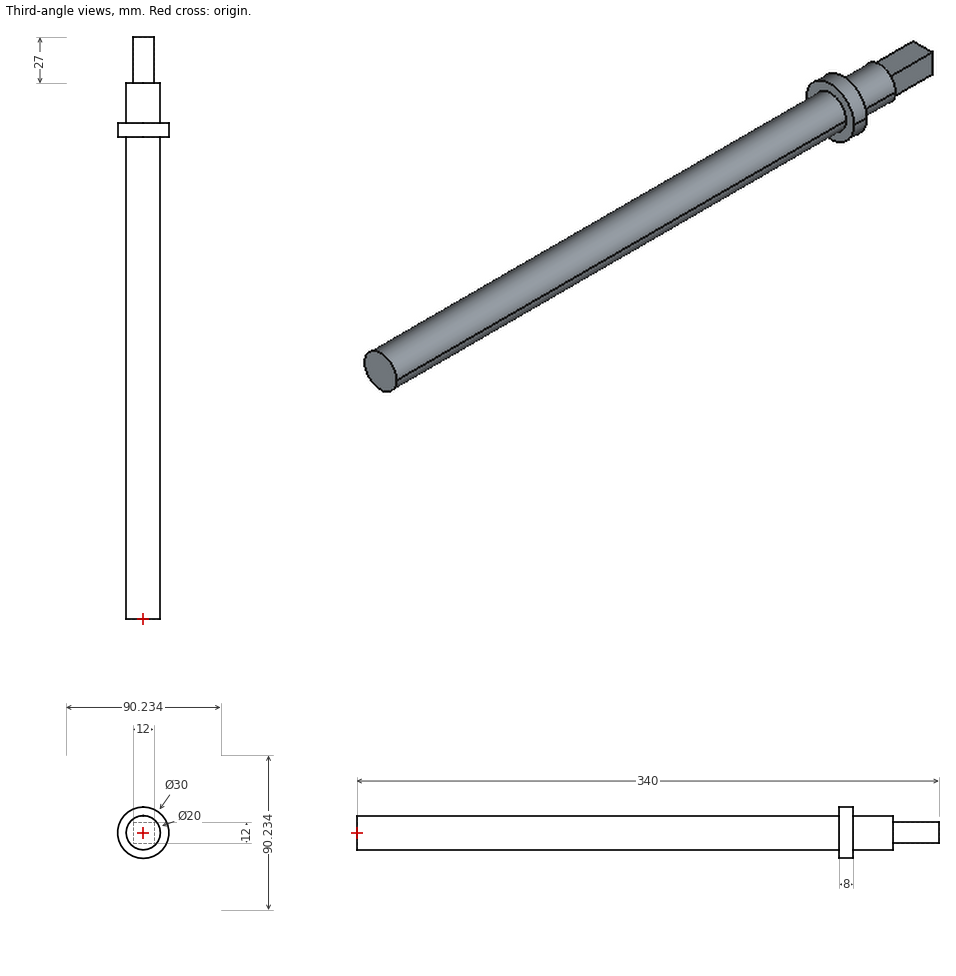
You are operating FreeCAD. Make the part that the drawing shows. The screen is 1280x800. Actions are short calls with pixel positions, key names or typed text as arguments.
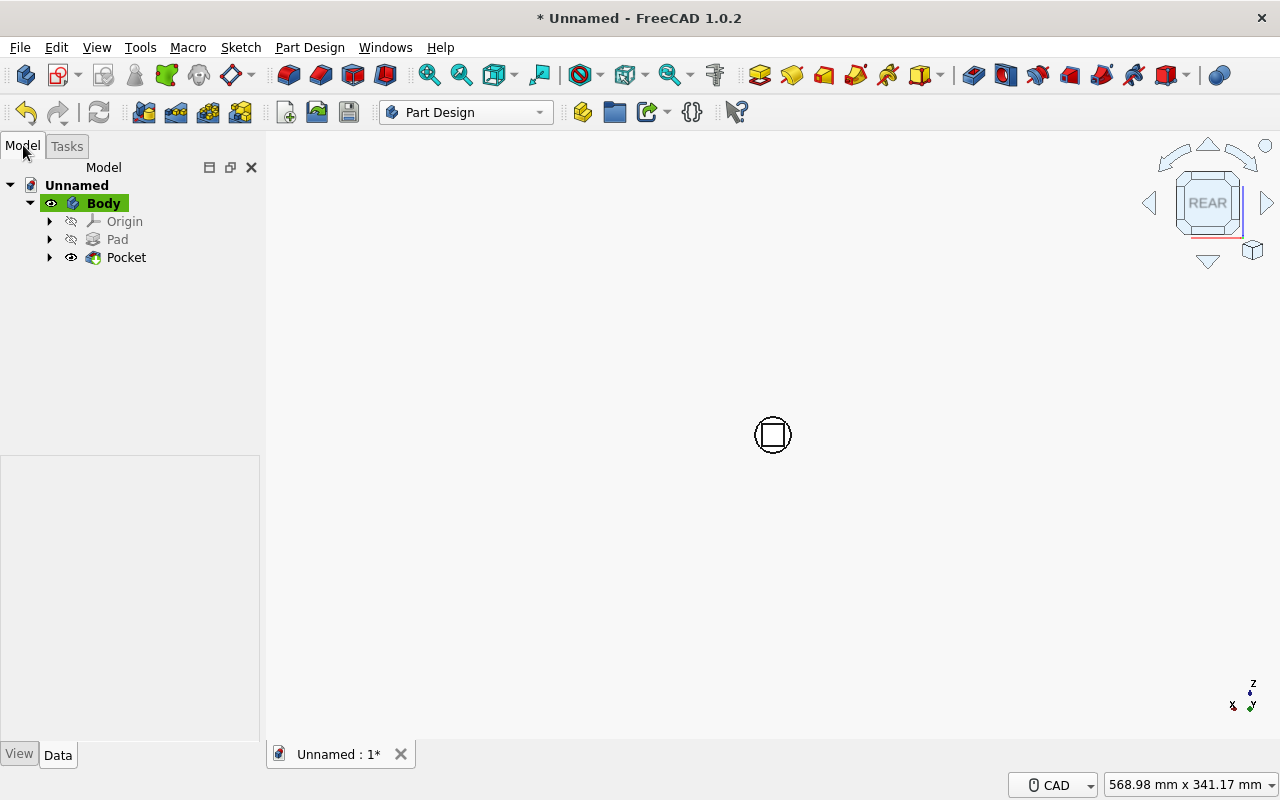
click(50, 221)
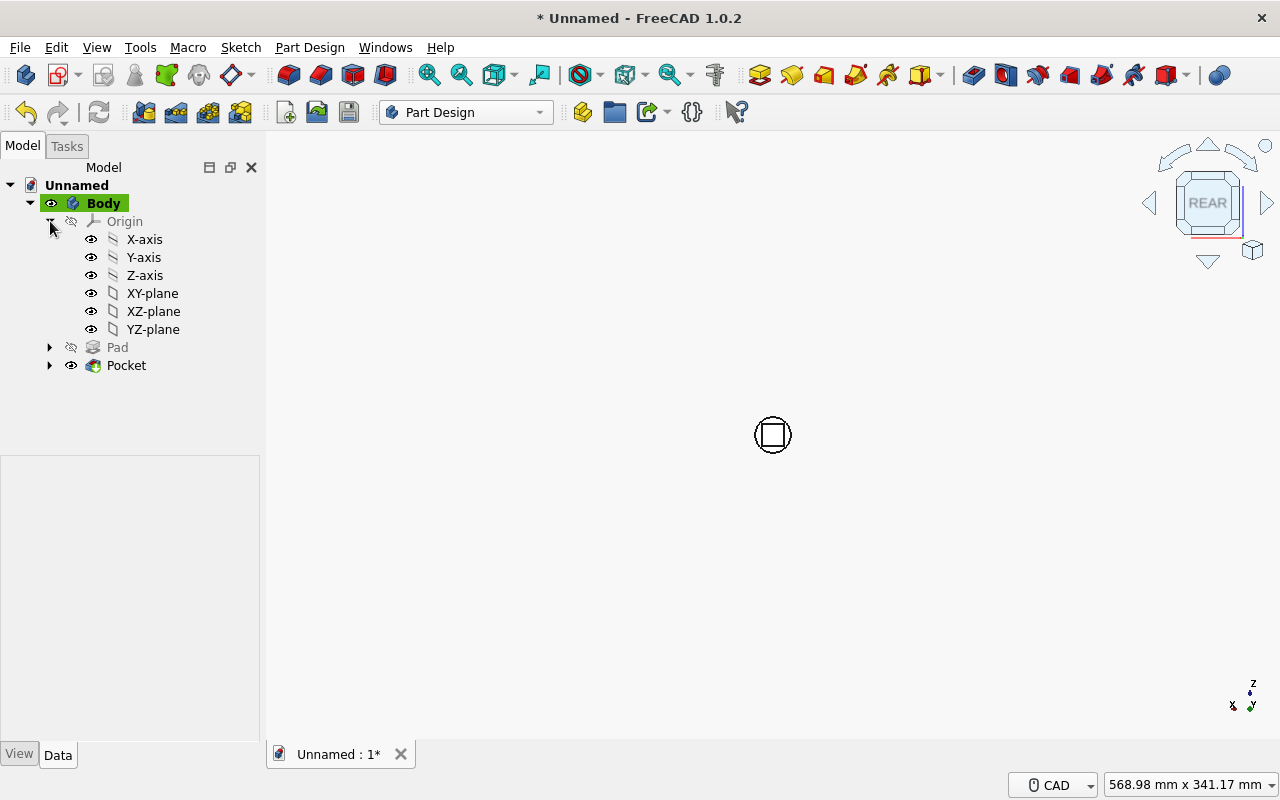
click(136, 311)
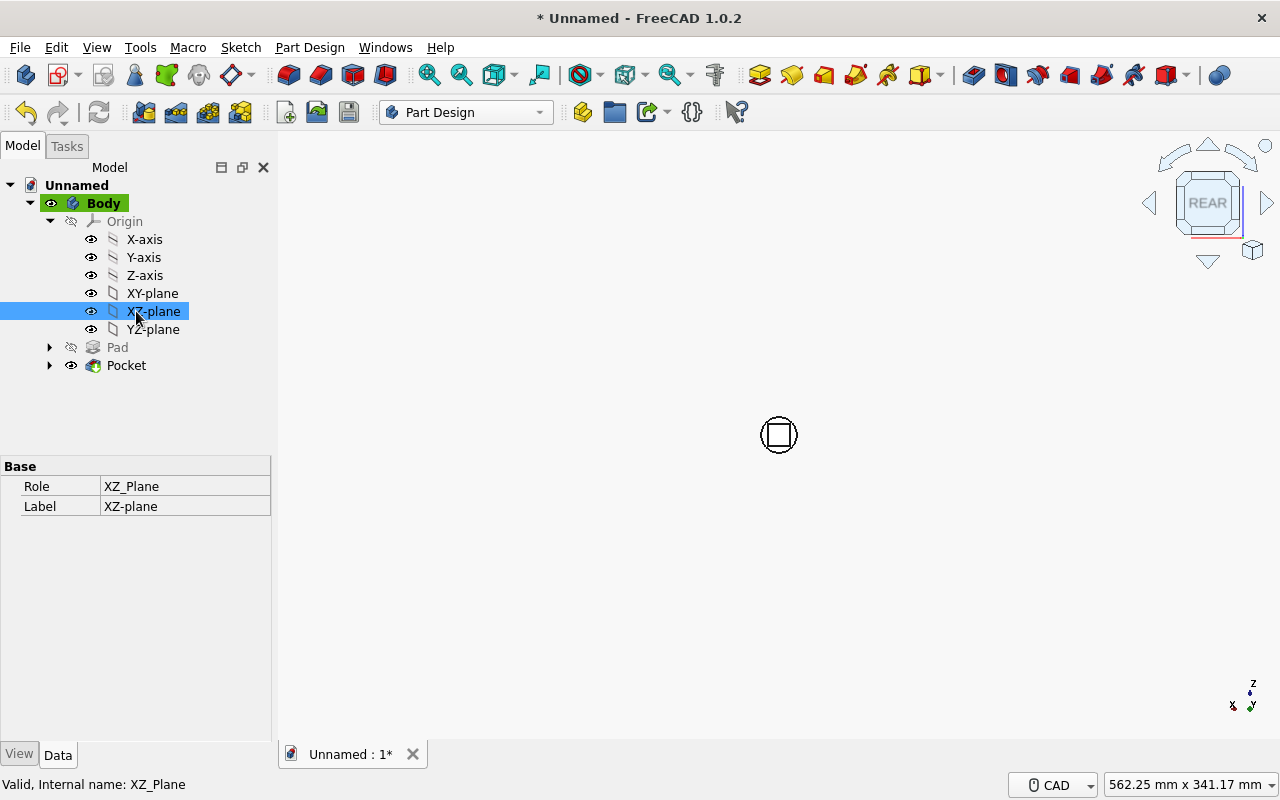
click(232, 76)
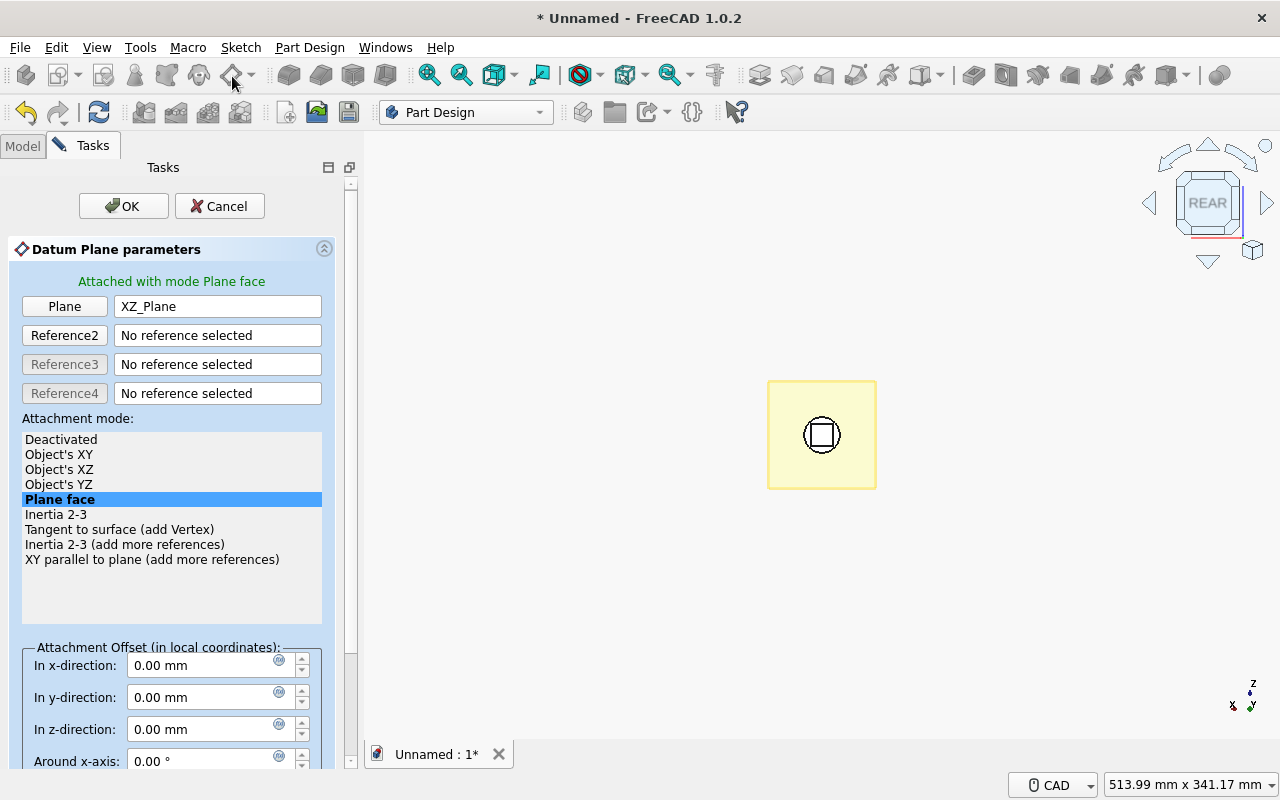
triple_click(210, 729)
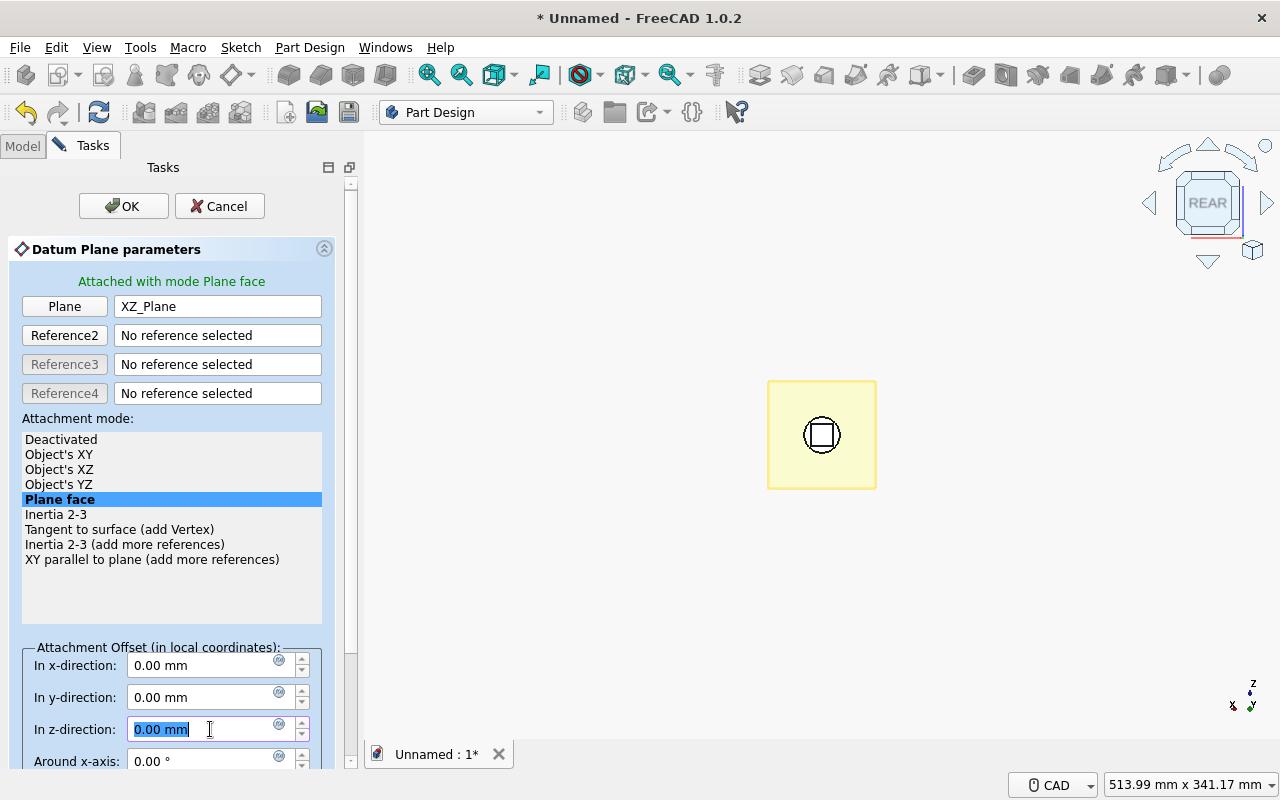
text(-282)
key(Tab)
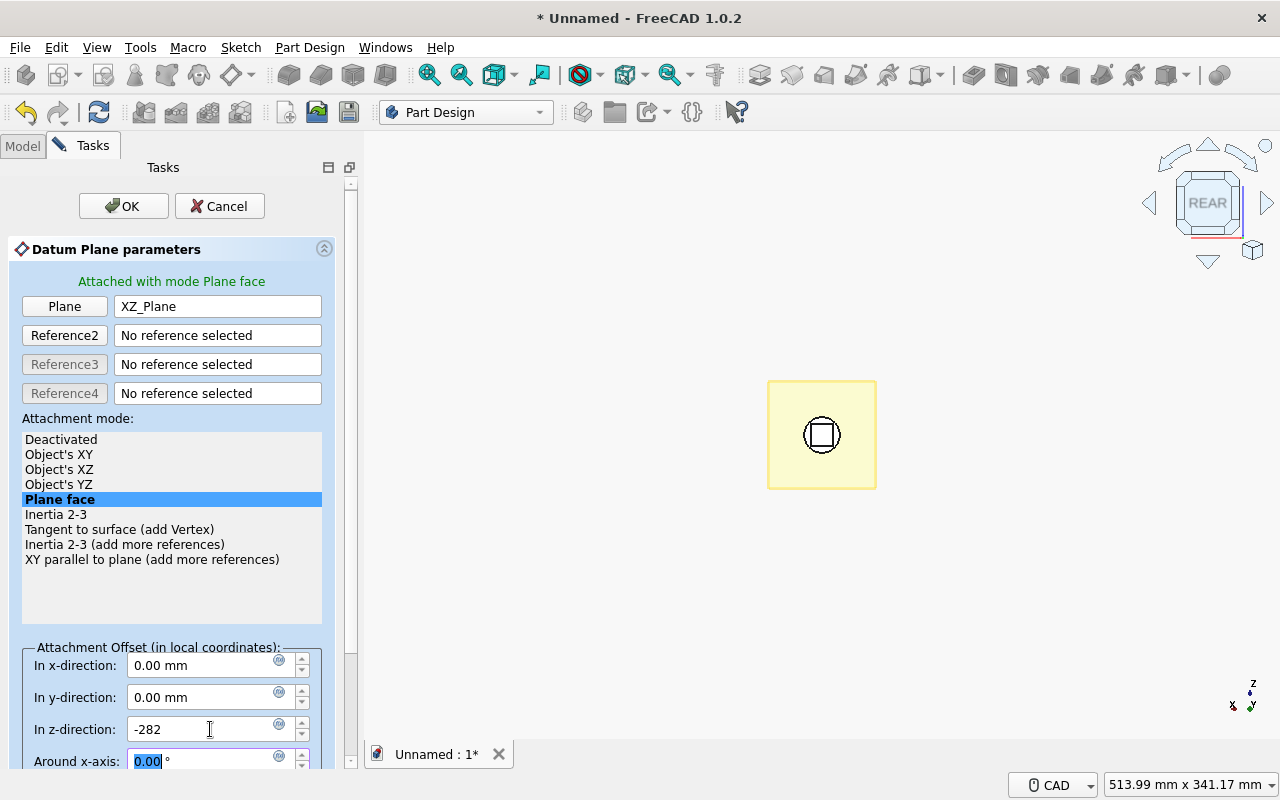
click(124, 206)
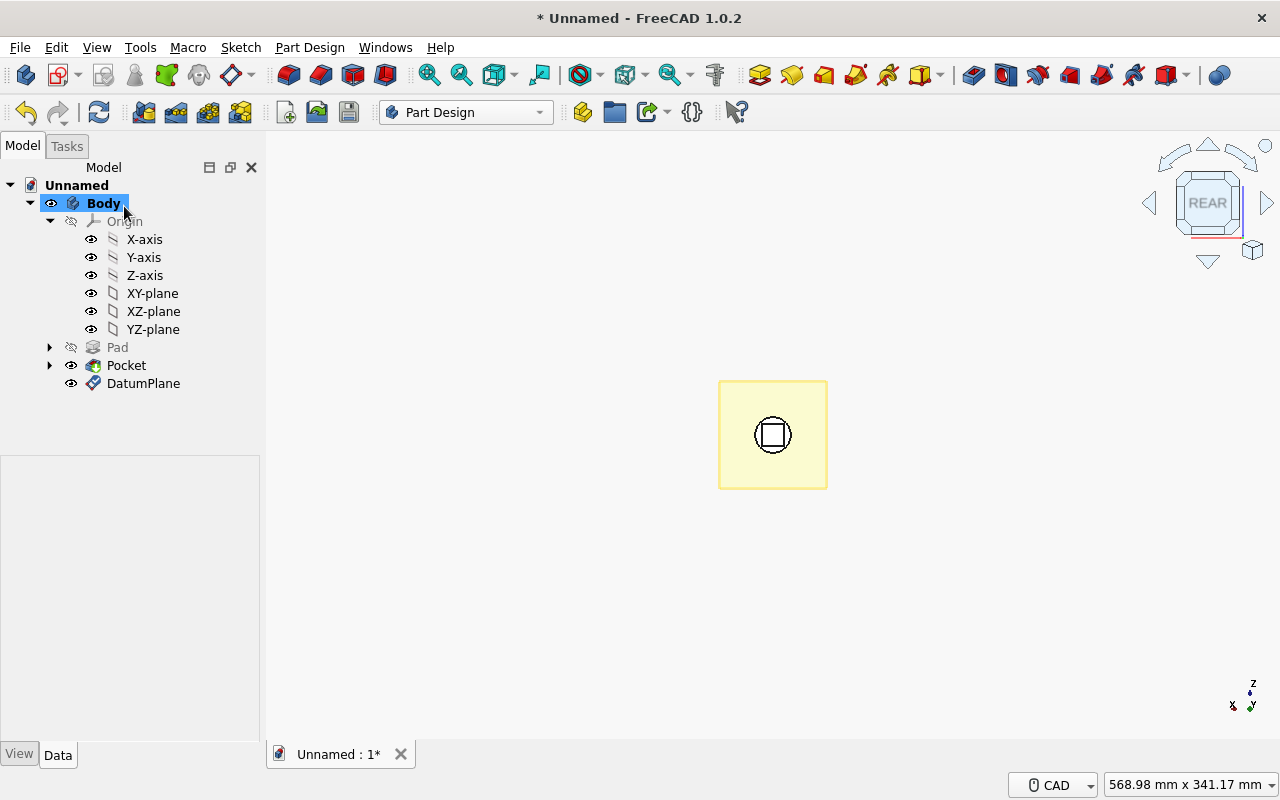
click(116, 383)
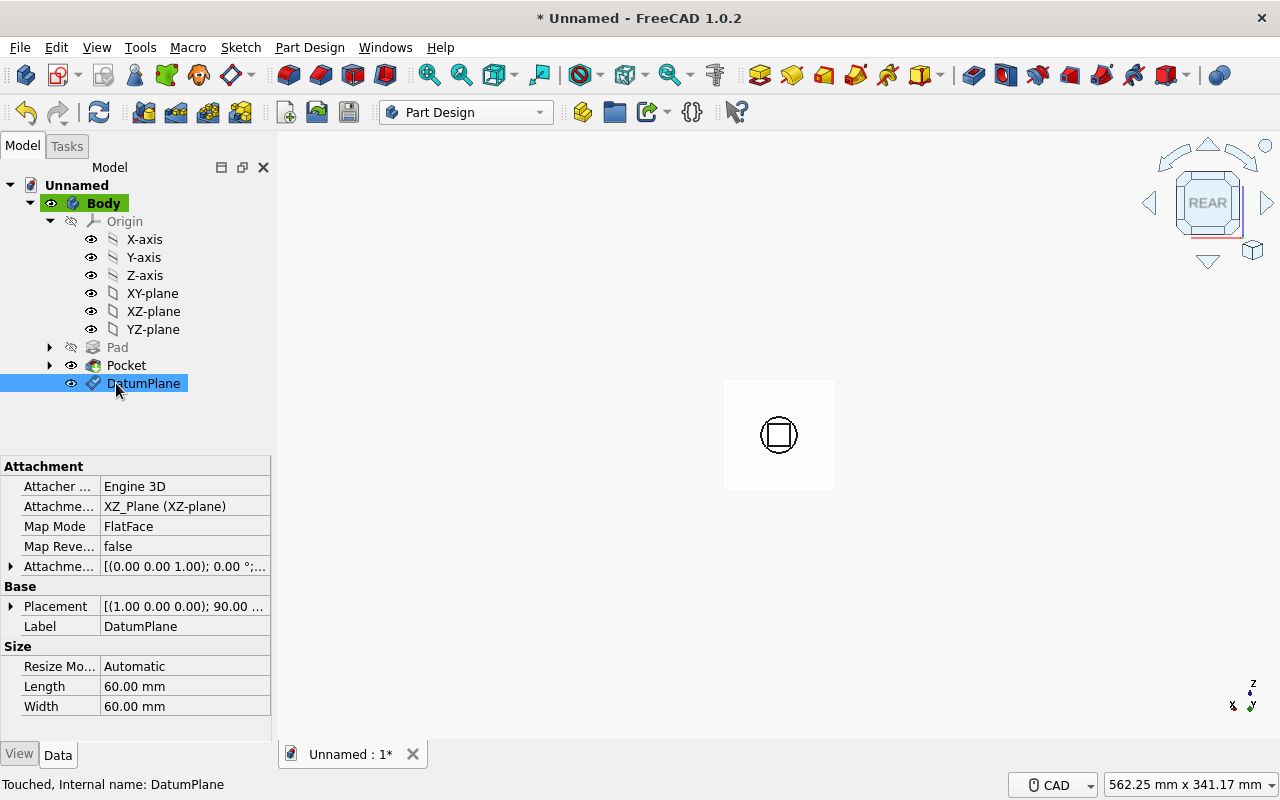
click(58, 76)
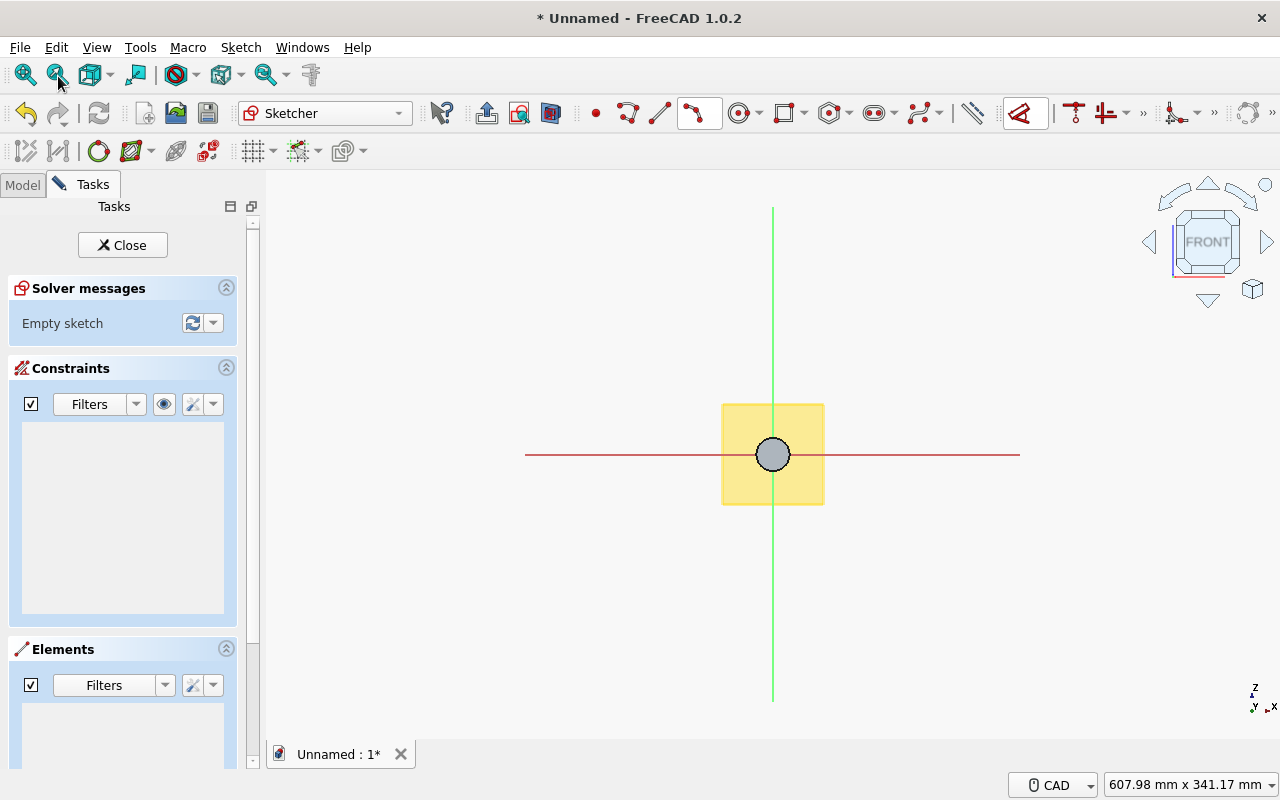
click(552, 114)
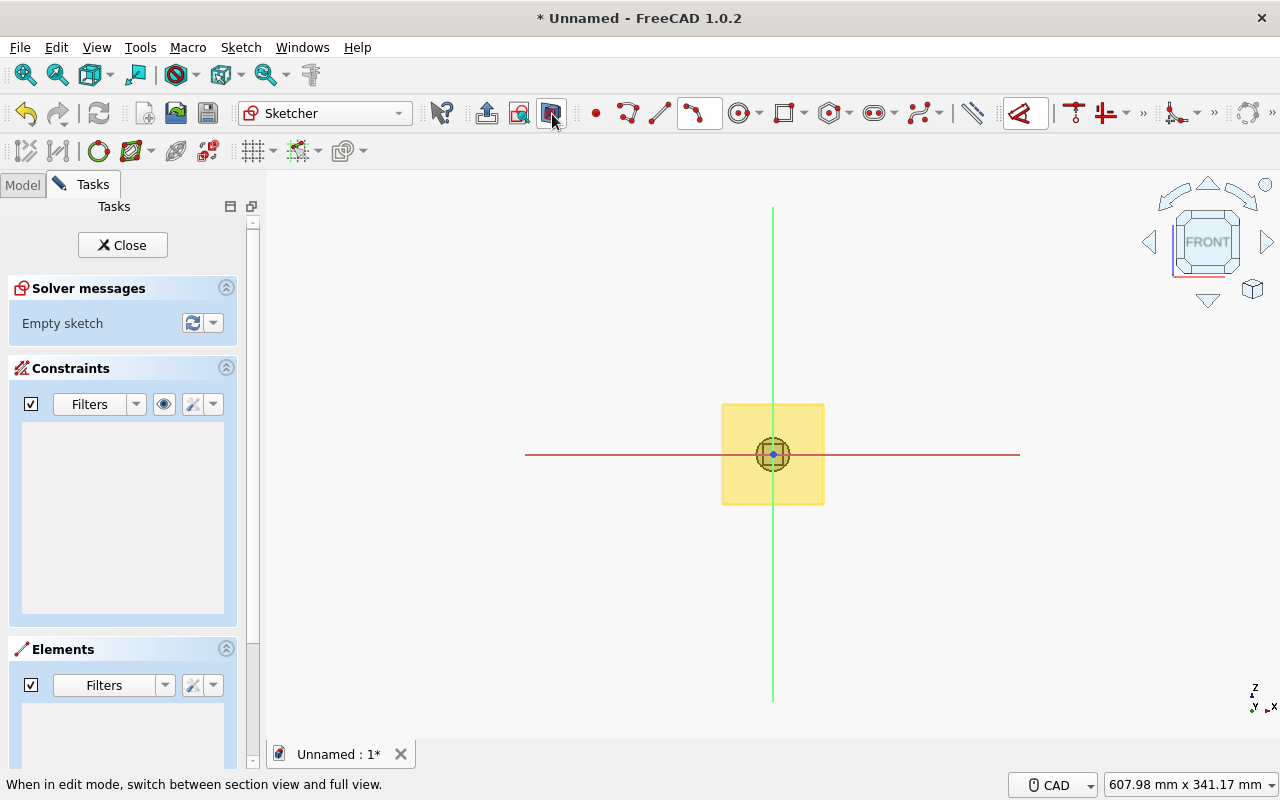
scroll(784, 455, up, 10)